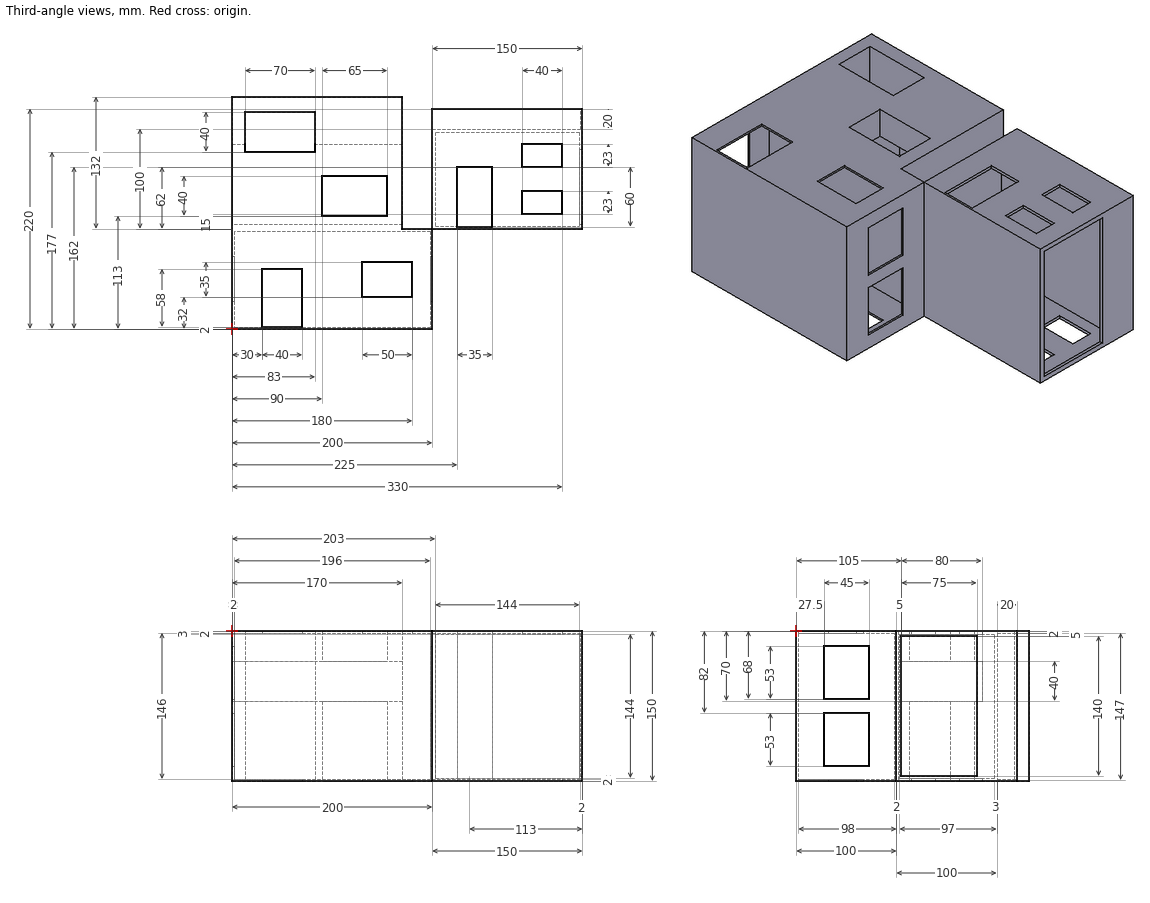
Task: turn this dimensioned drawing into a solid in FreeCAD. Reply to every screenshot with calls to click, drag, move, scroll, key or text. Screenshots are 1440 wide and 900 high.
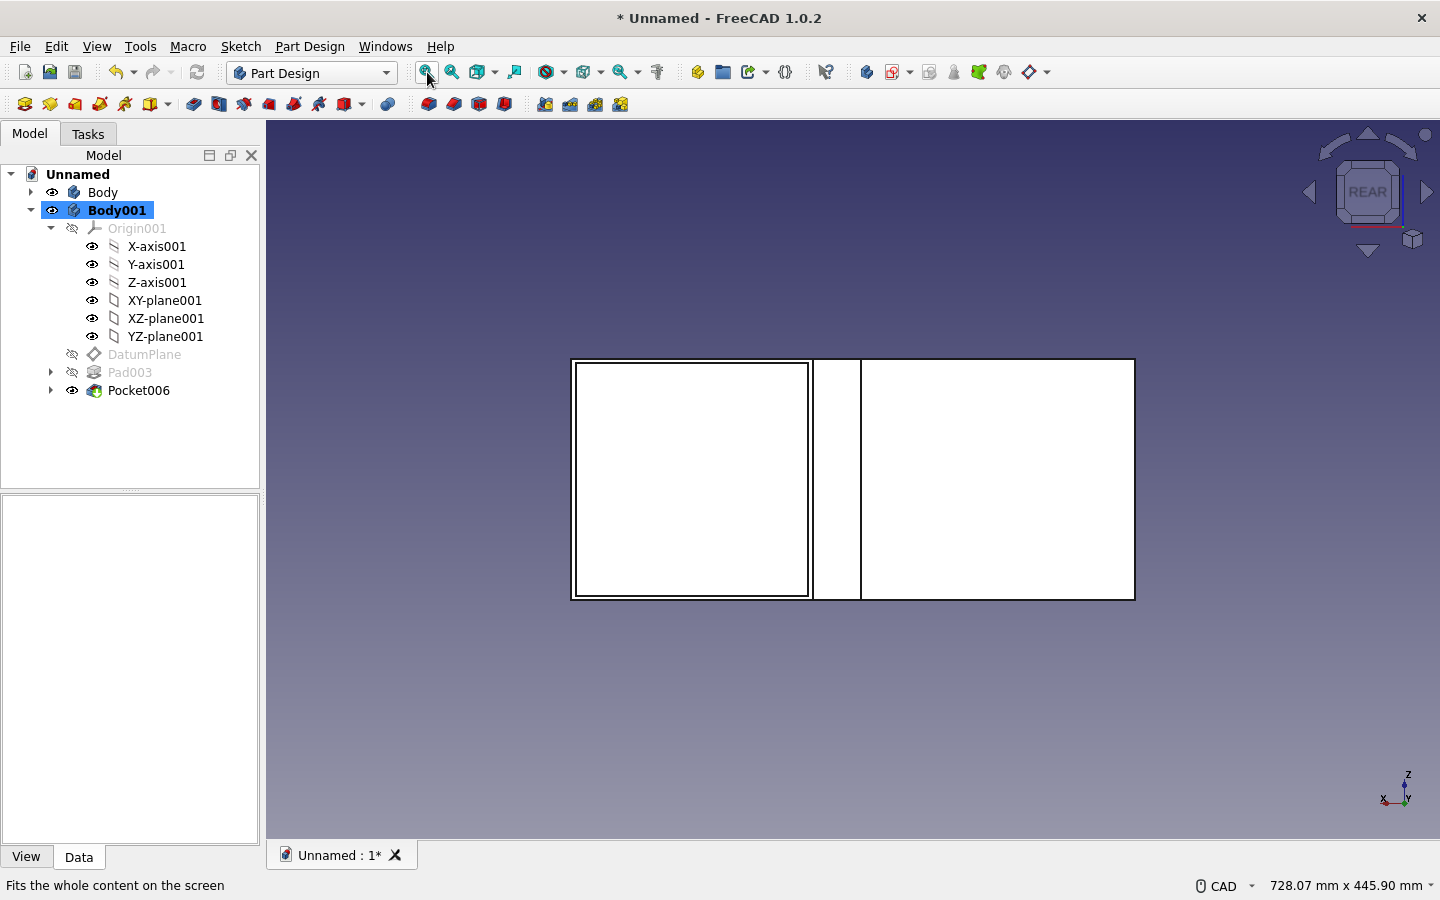
scroll(572, 517, up, 11)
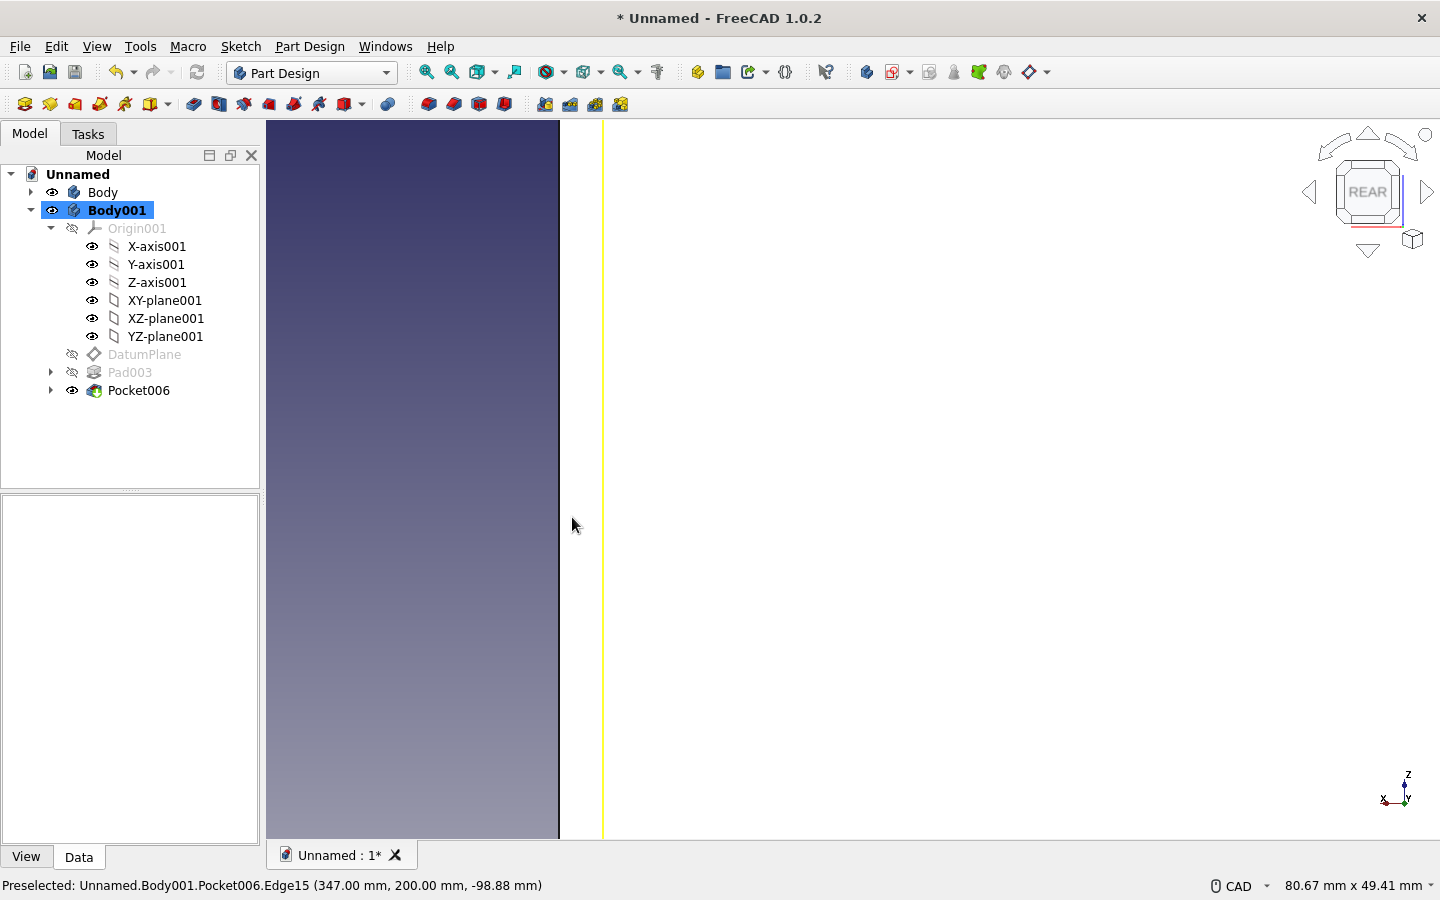
click(574, 522)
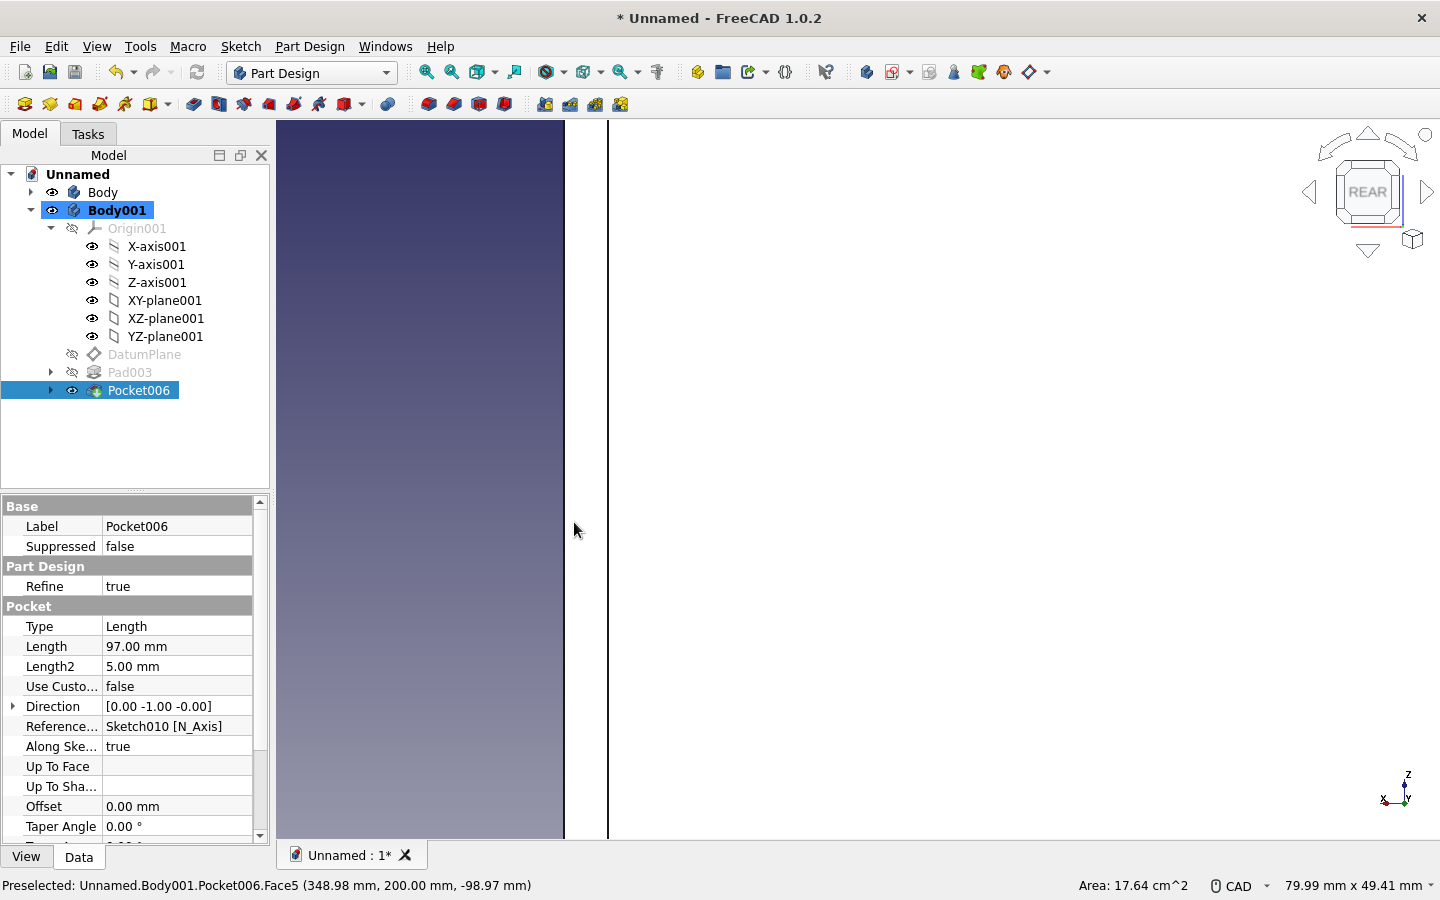
click(892, 72)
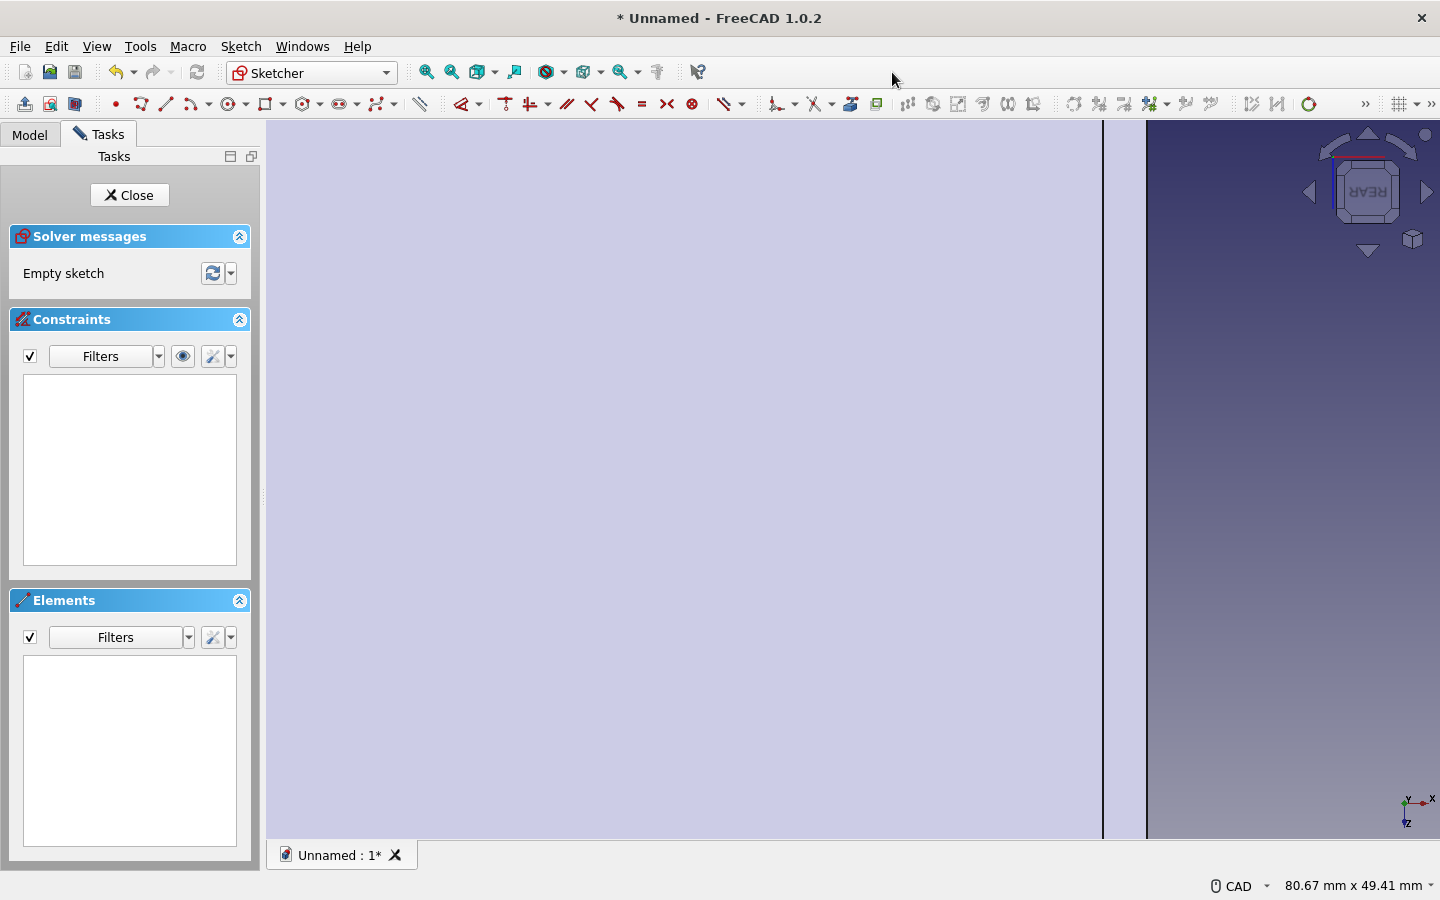
scroll(1126, 432, down, 10)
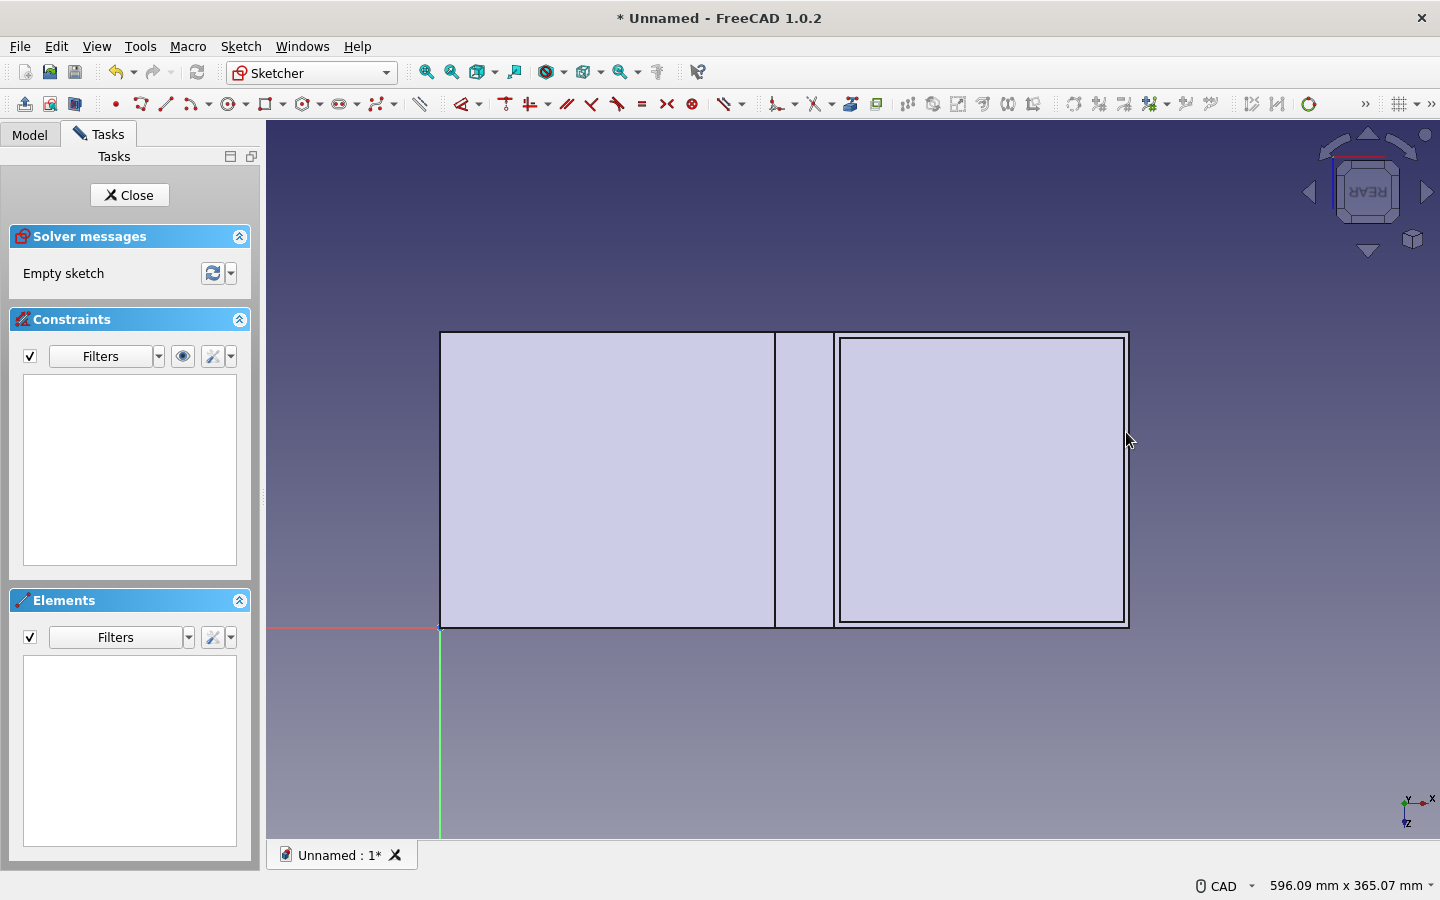
click(264, 104)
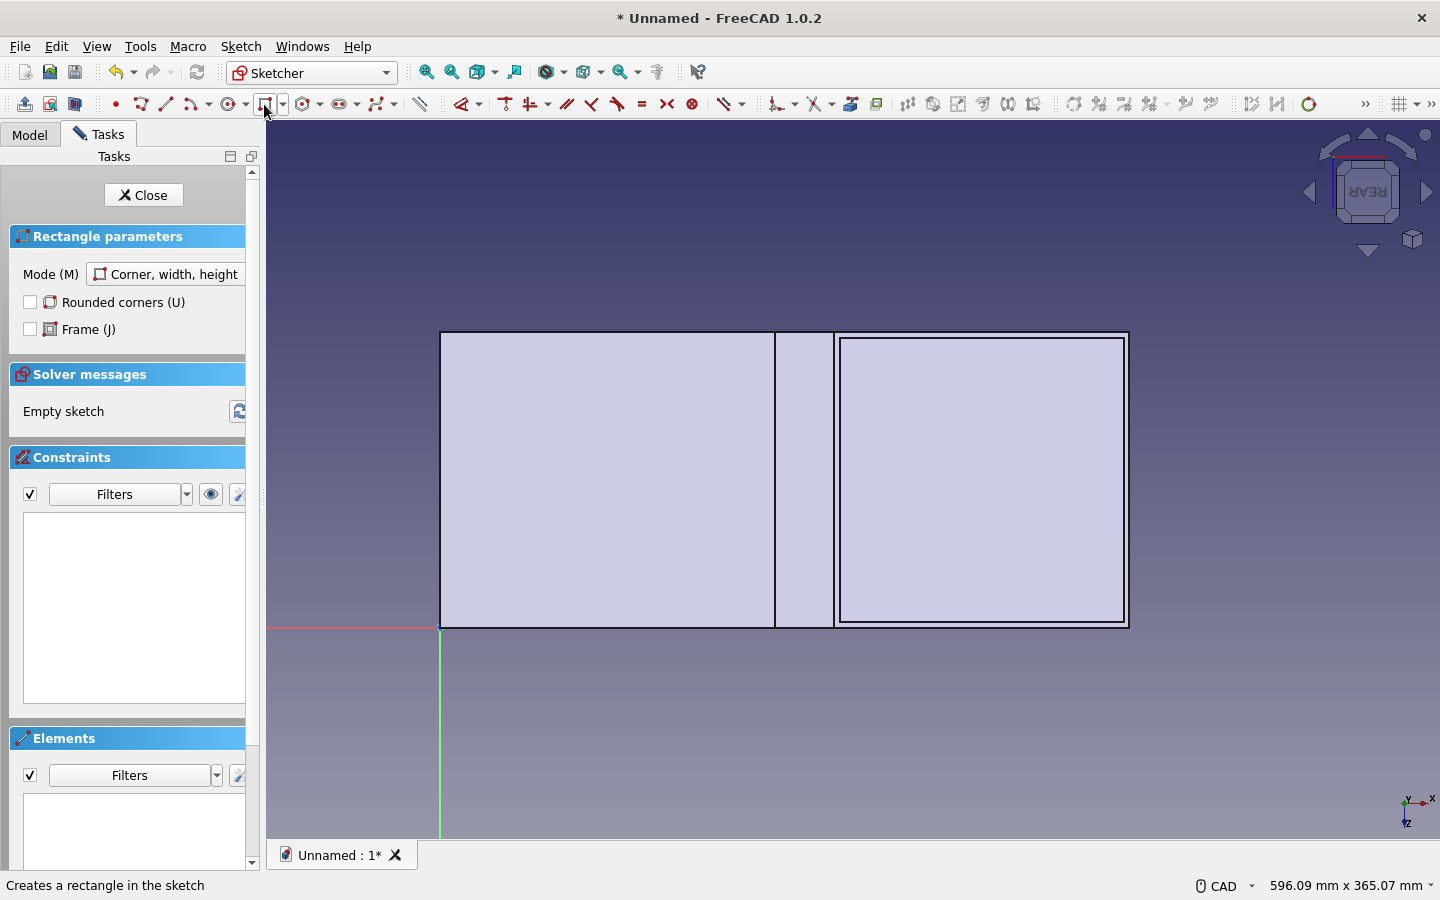
click(834, 332)
click(1129, 628)
key(Escape)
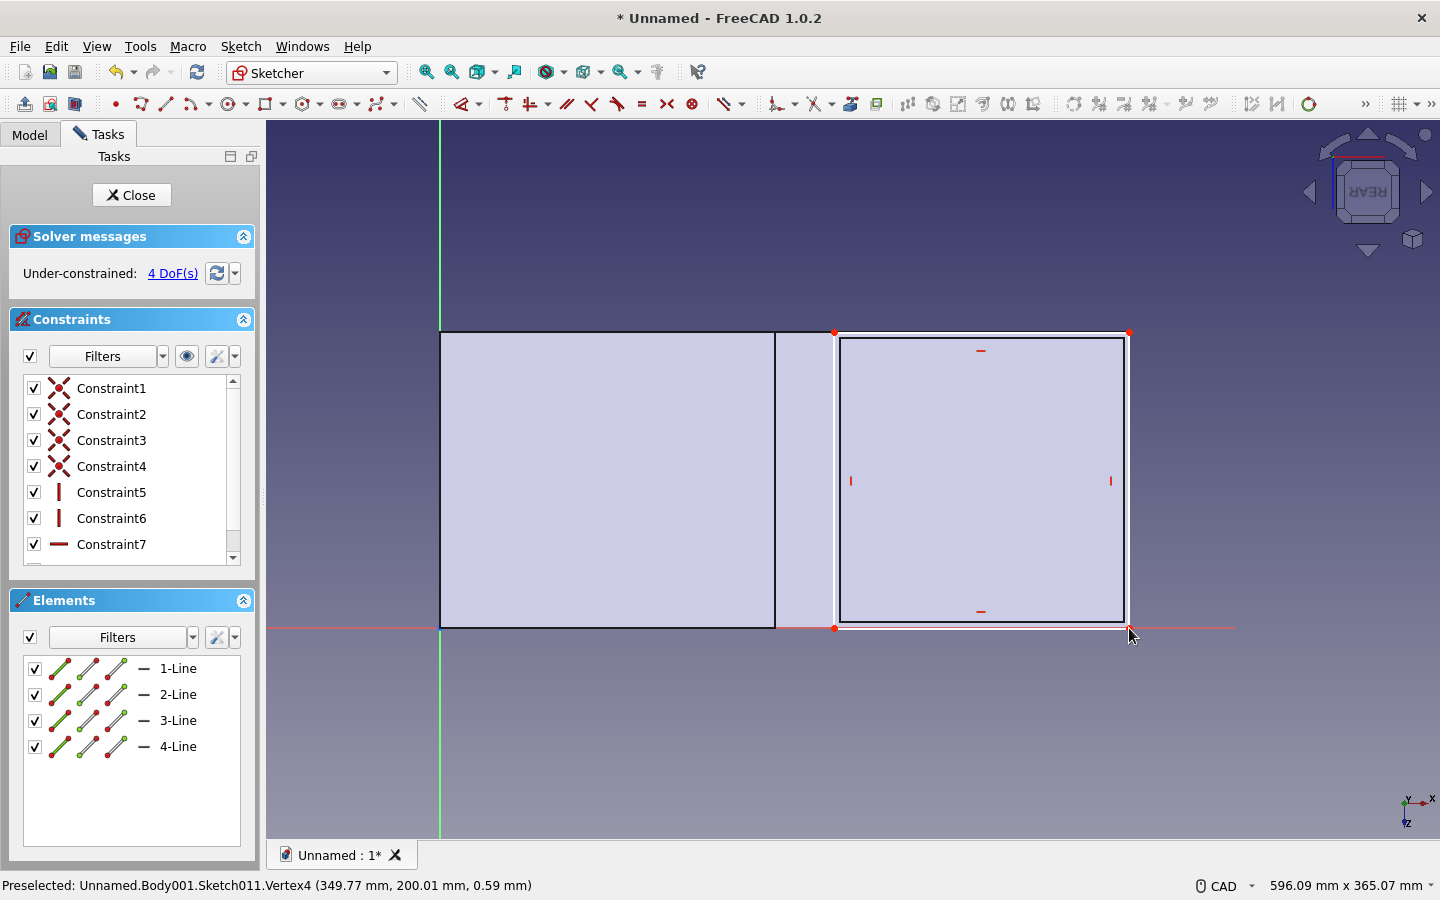
click(834, 629)